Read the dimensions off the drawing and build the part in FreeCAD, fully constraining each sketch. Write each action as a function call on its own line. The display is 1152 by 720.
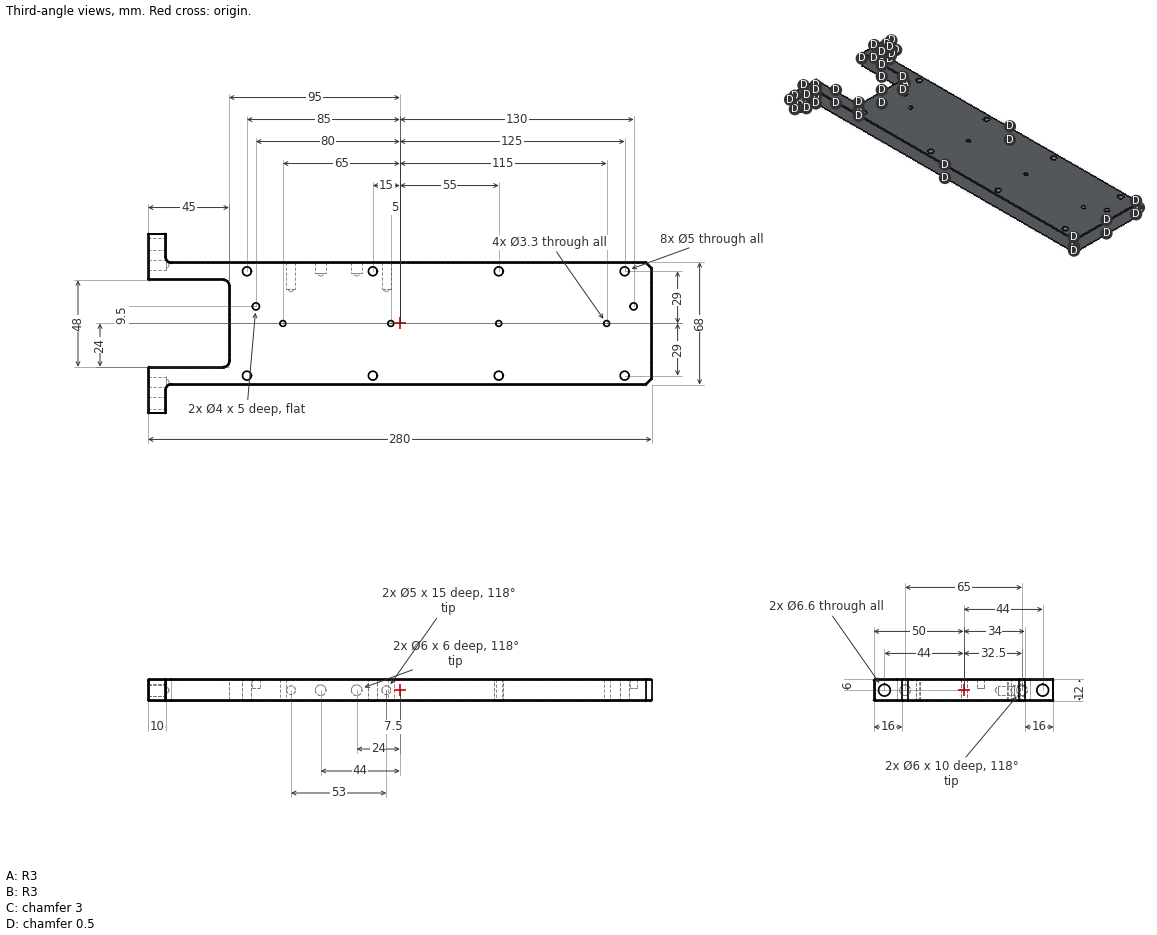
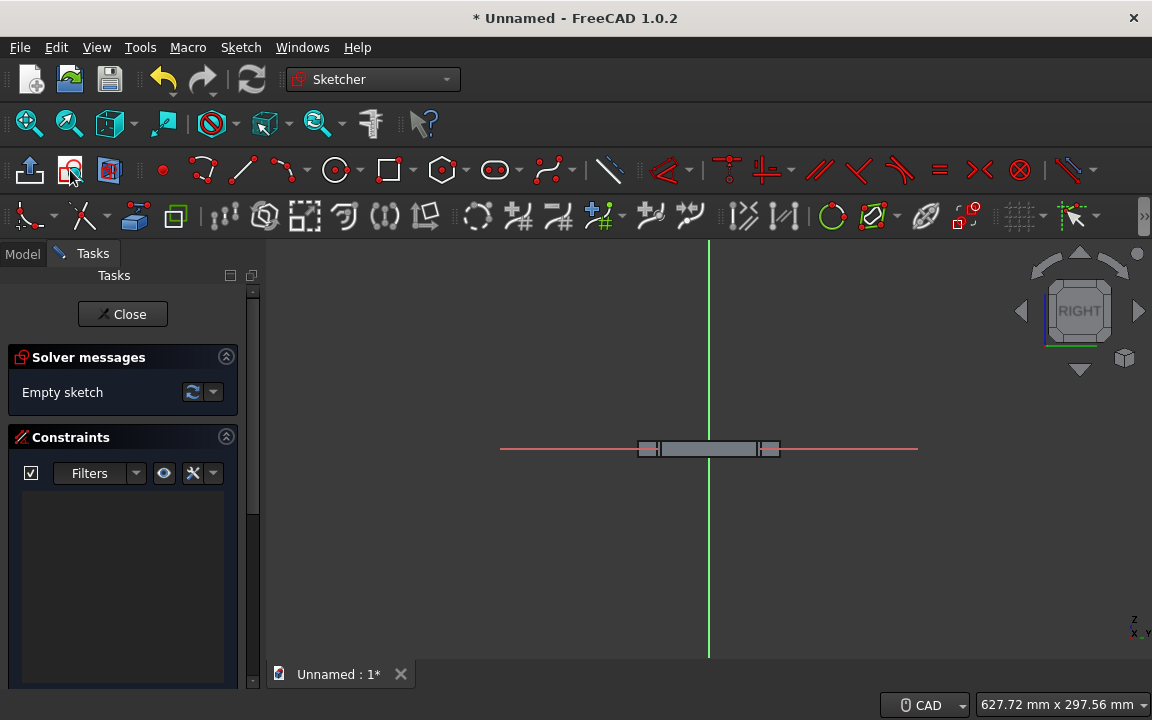
click(110, 170)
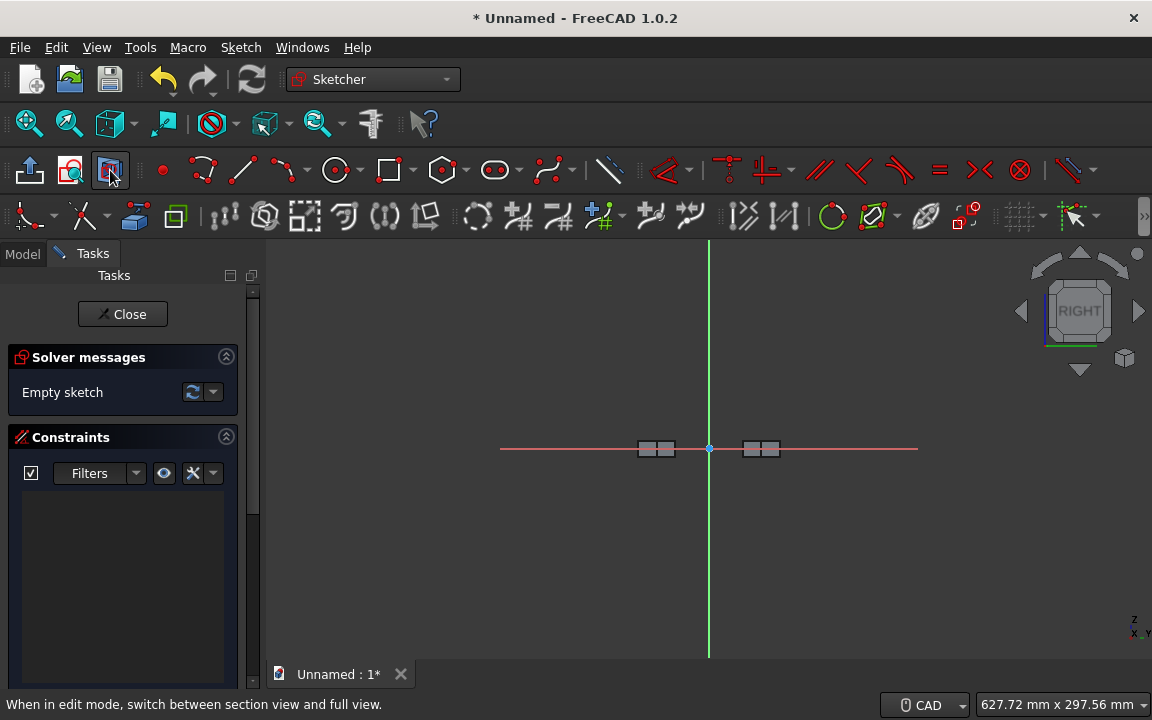
scroll(739, 449, up, 6)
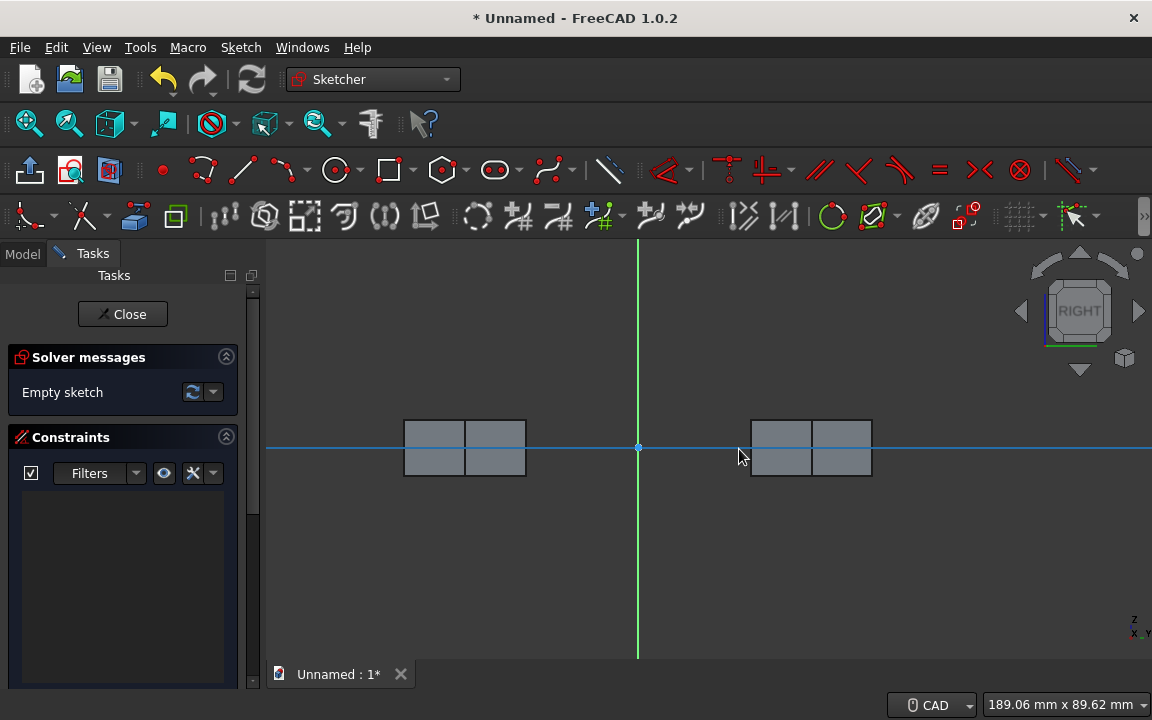
key(g)
key(c)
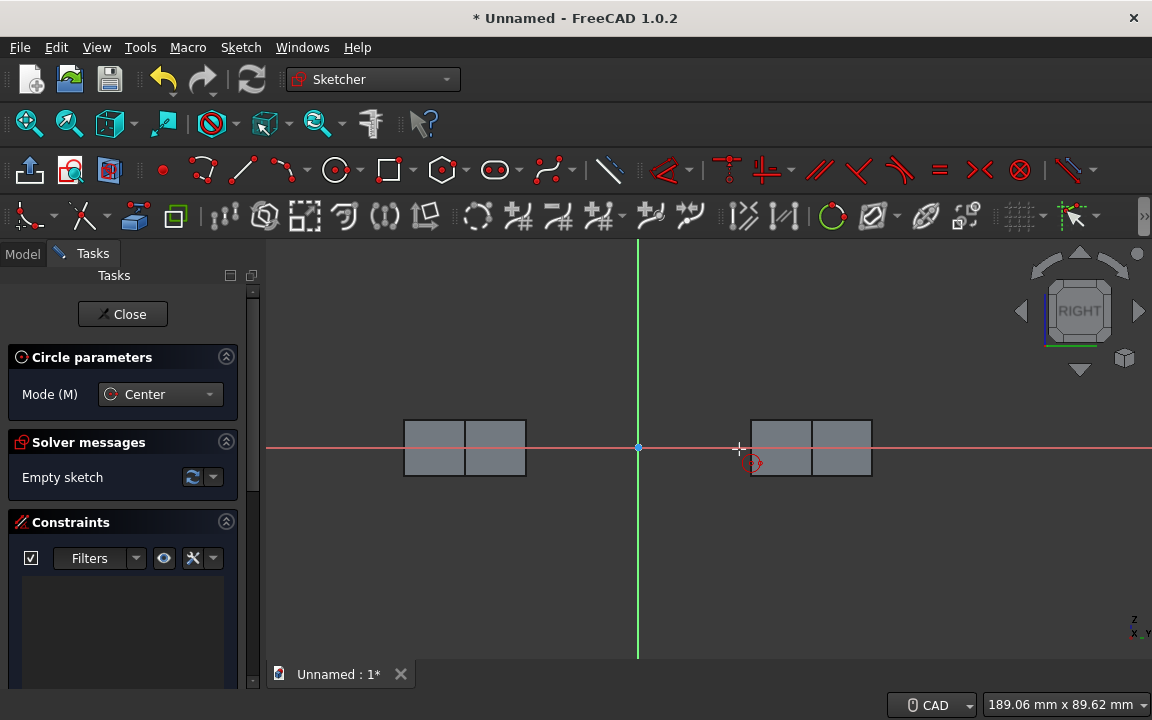
scroll(432, 448, up, 2)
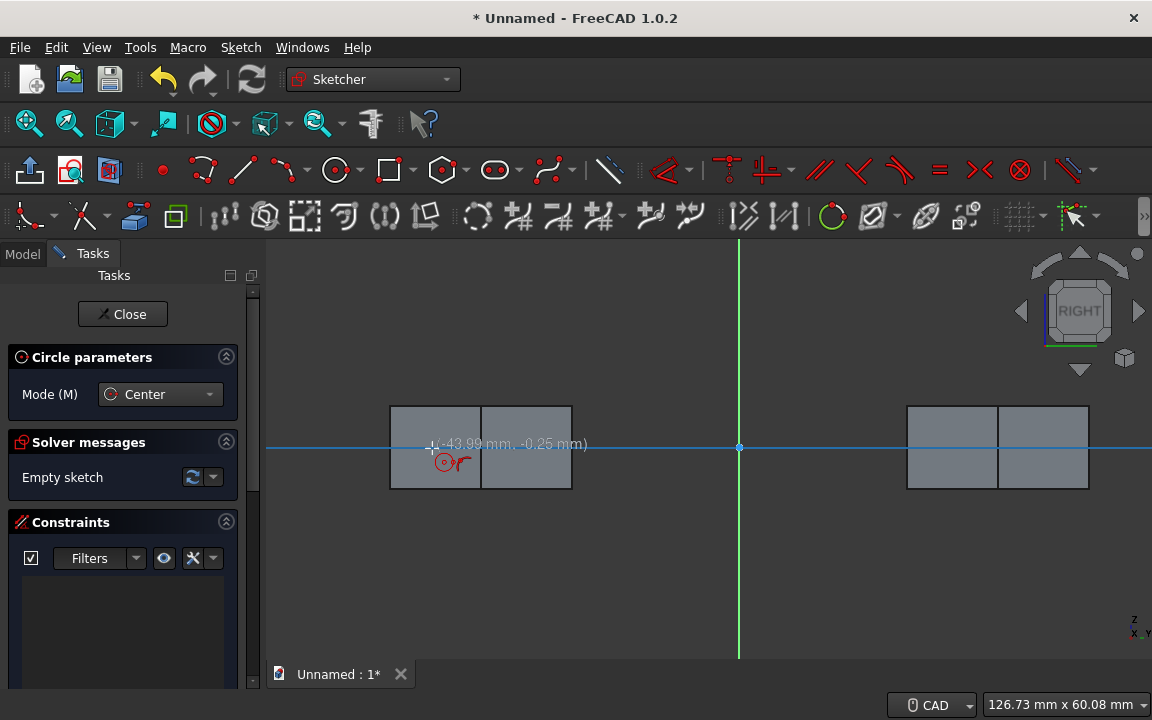
click(432, 448)
move(448, 431)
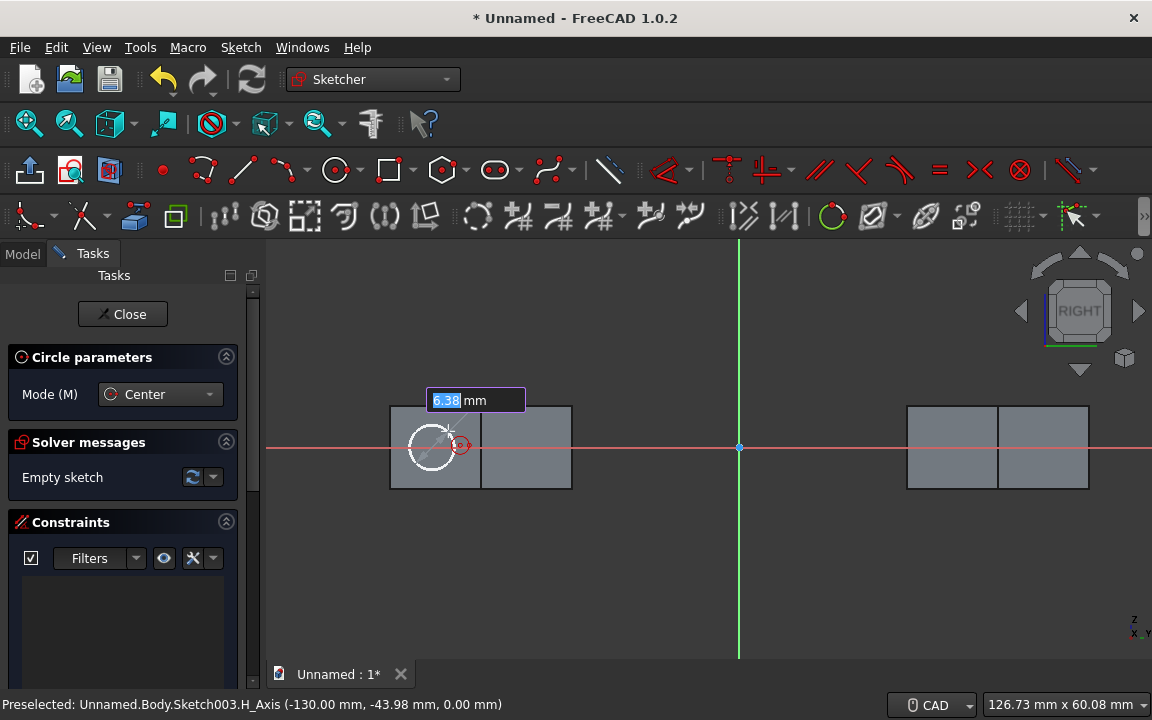
text(6.6)
key(Return)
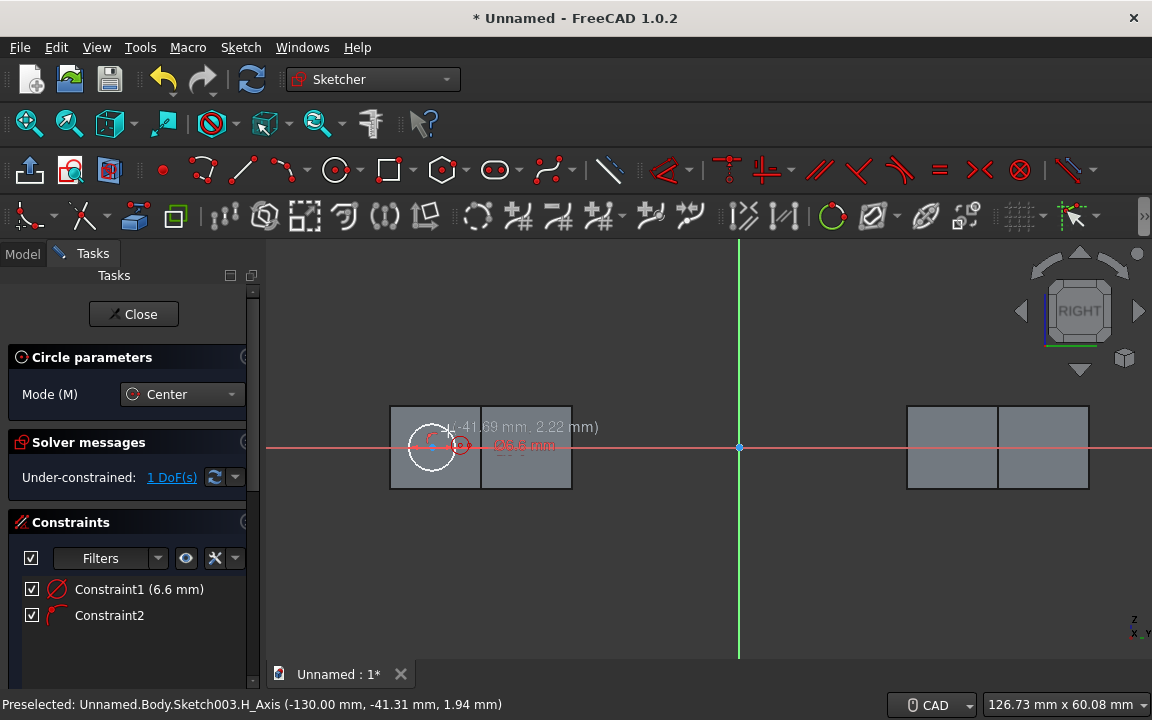
scroll(439, 452, down, 2)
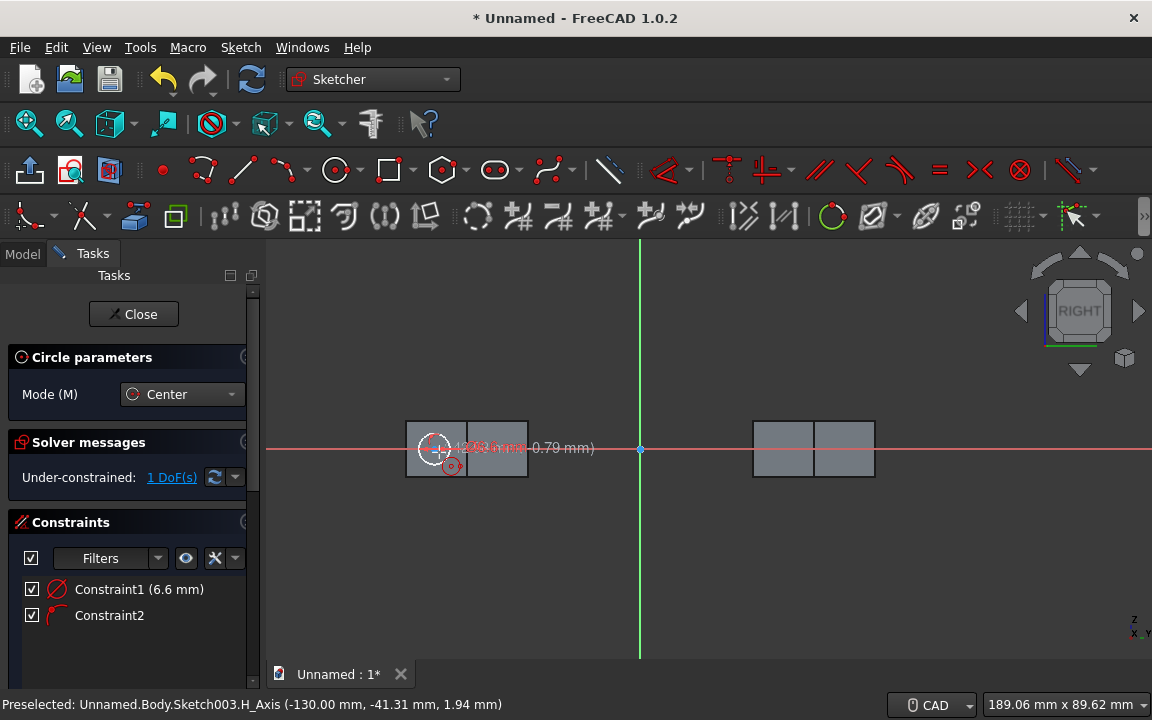
scroll(847, 449, up, 2)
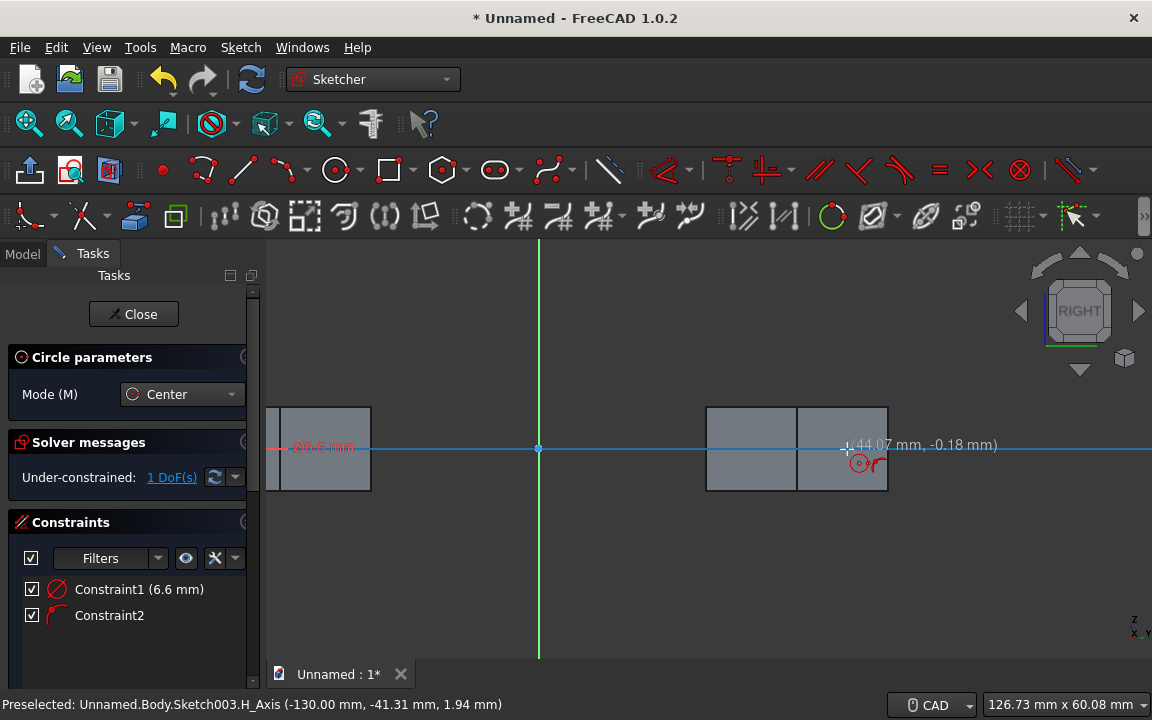
click(846, 449)
move(862, 433)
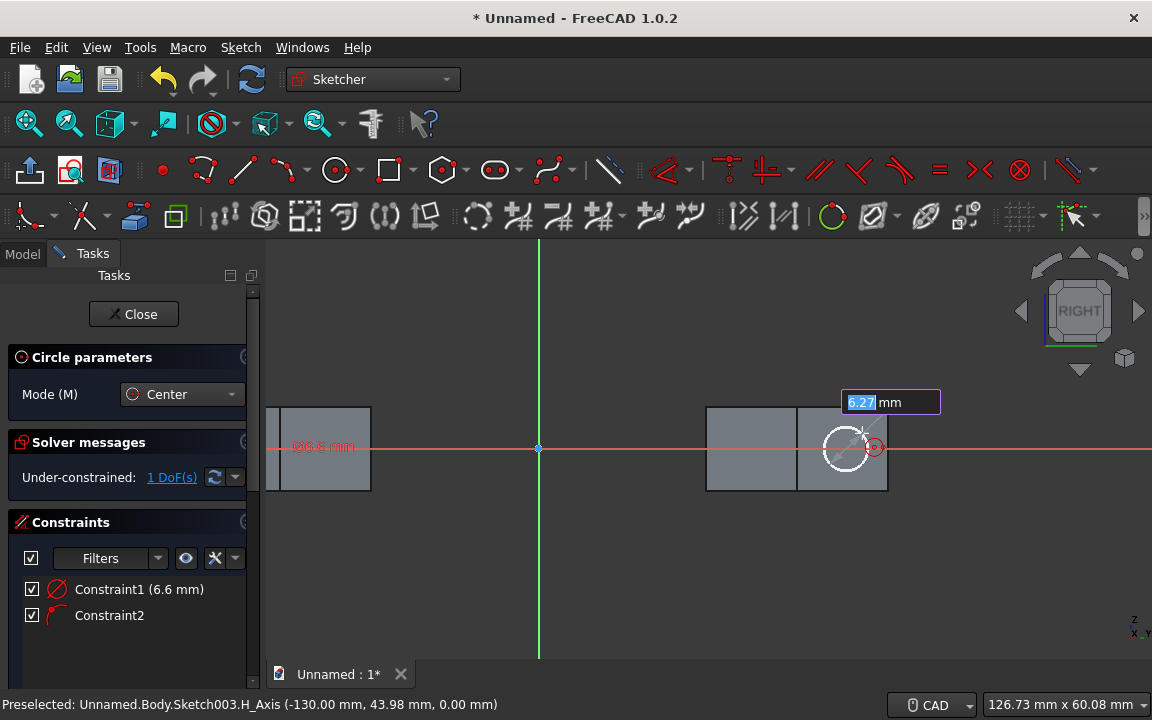
text(6.6)
key(Return)
key(Escape)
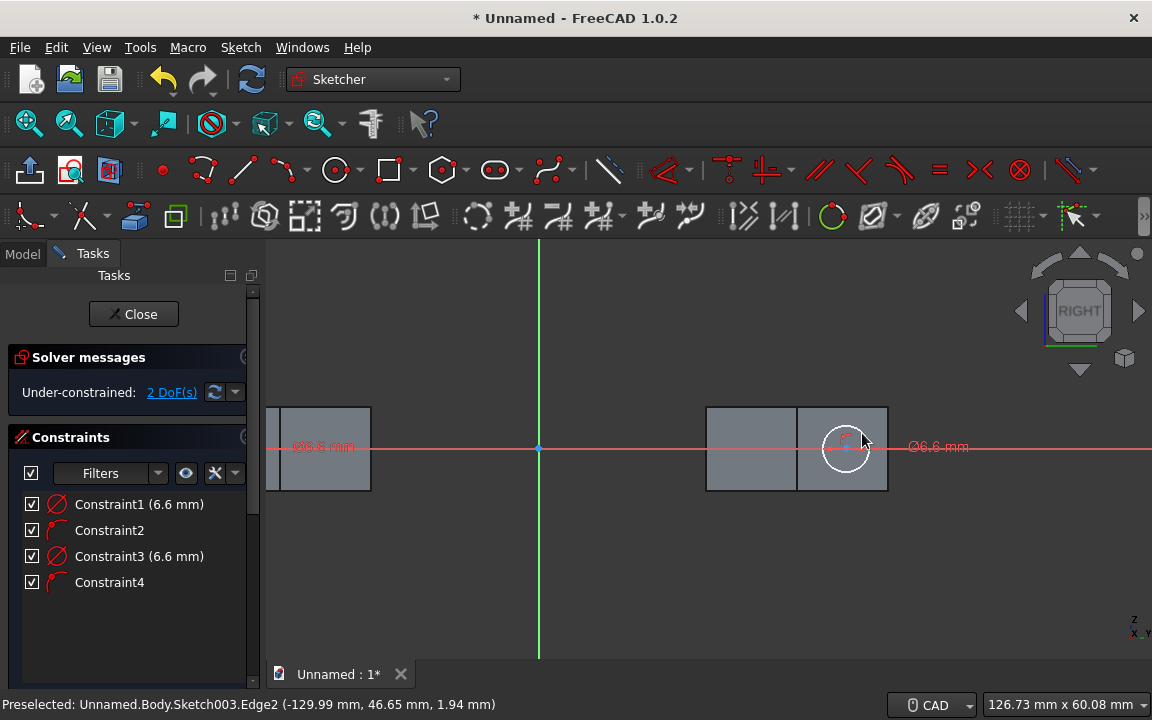
key(d)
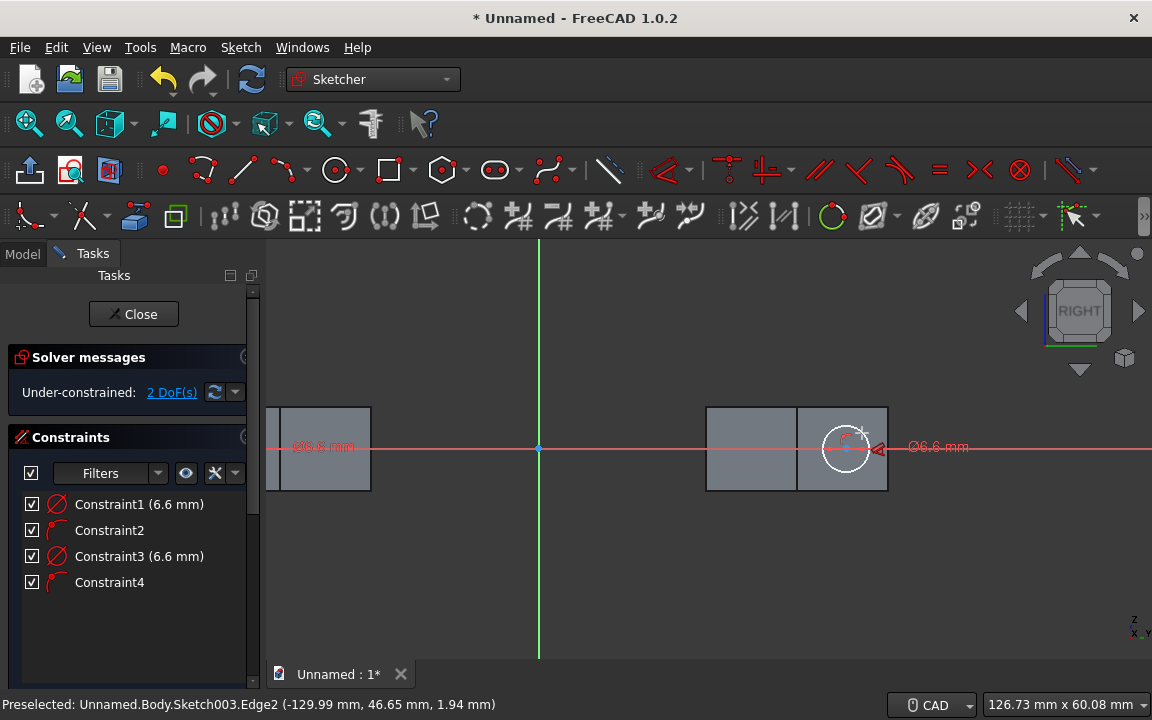
scroll(848, 449, down, 2)